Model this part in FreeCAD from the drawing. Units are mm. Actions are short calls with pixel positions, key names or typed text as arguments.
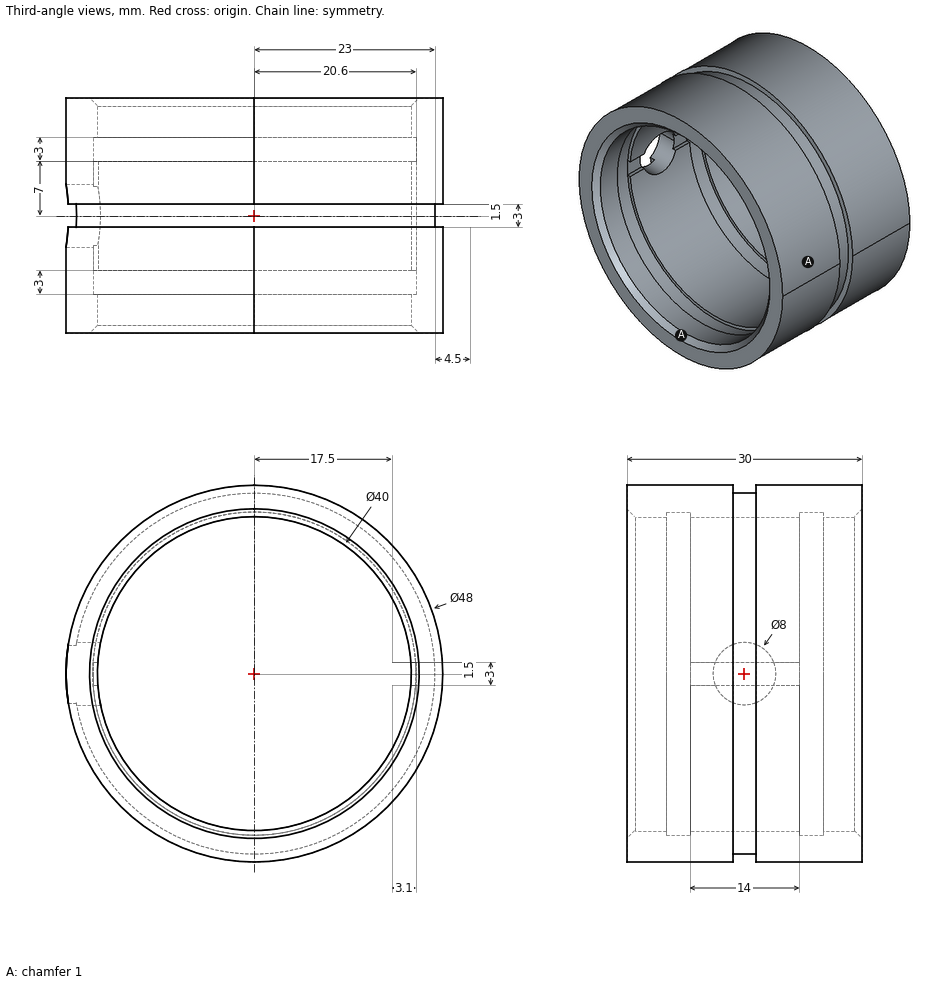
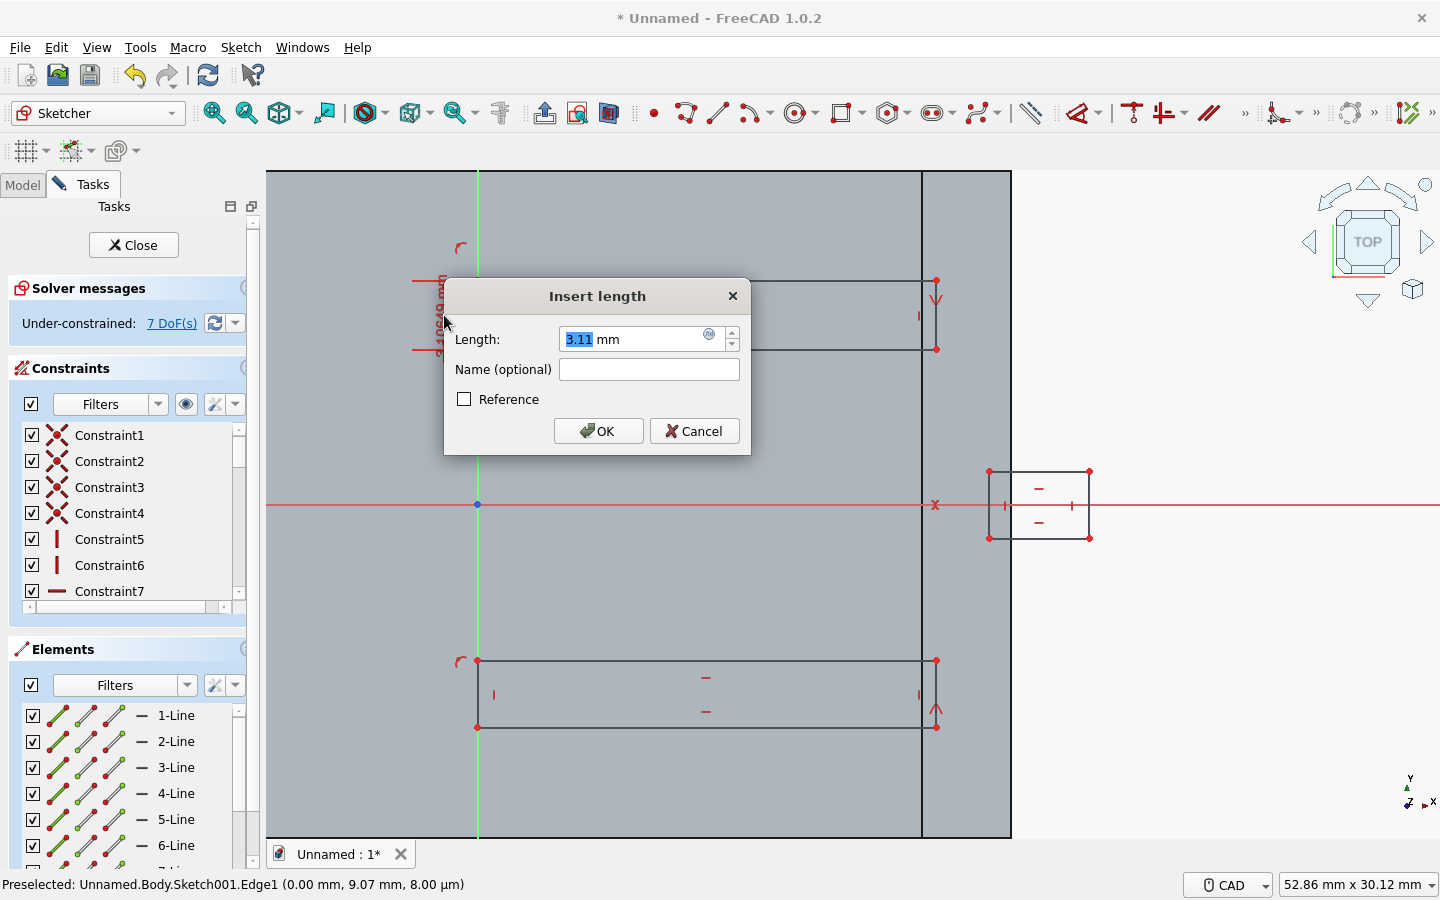
text(3)
key(Return)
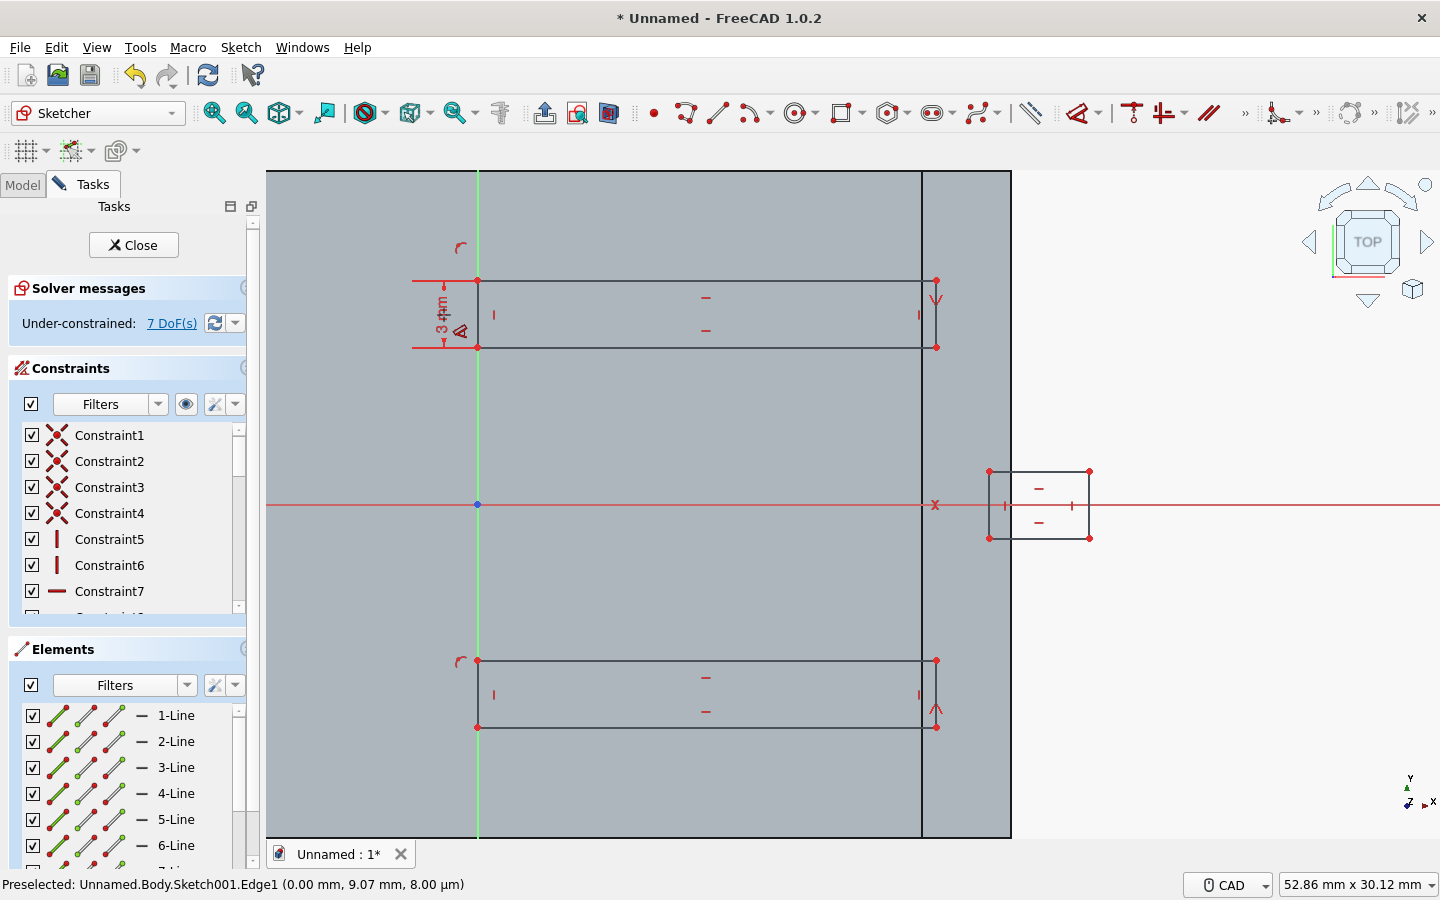
click(478, 681)
click(444, 695)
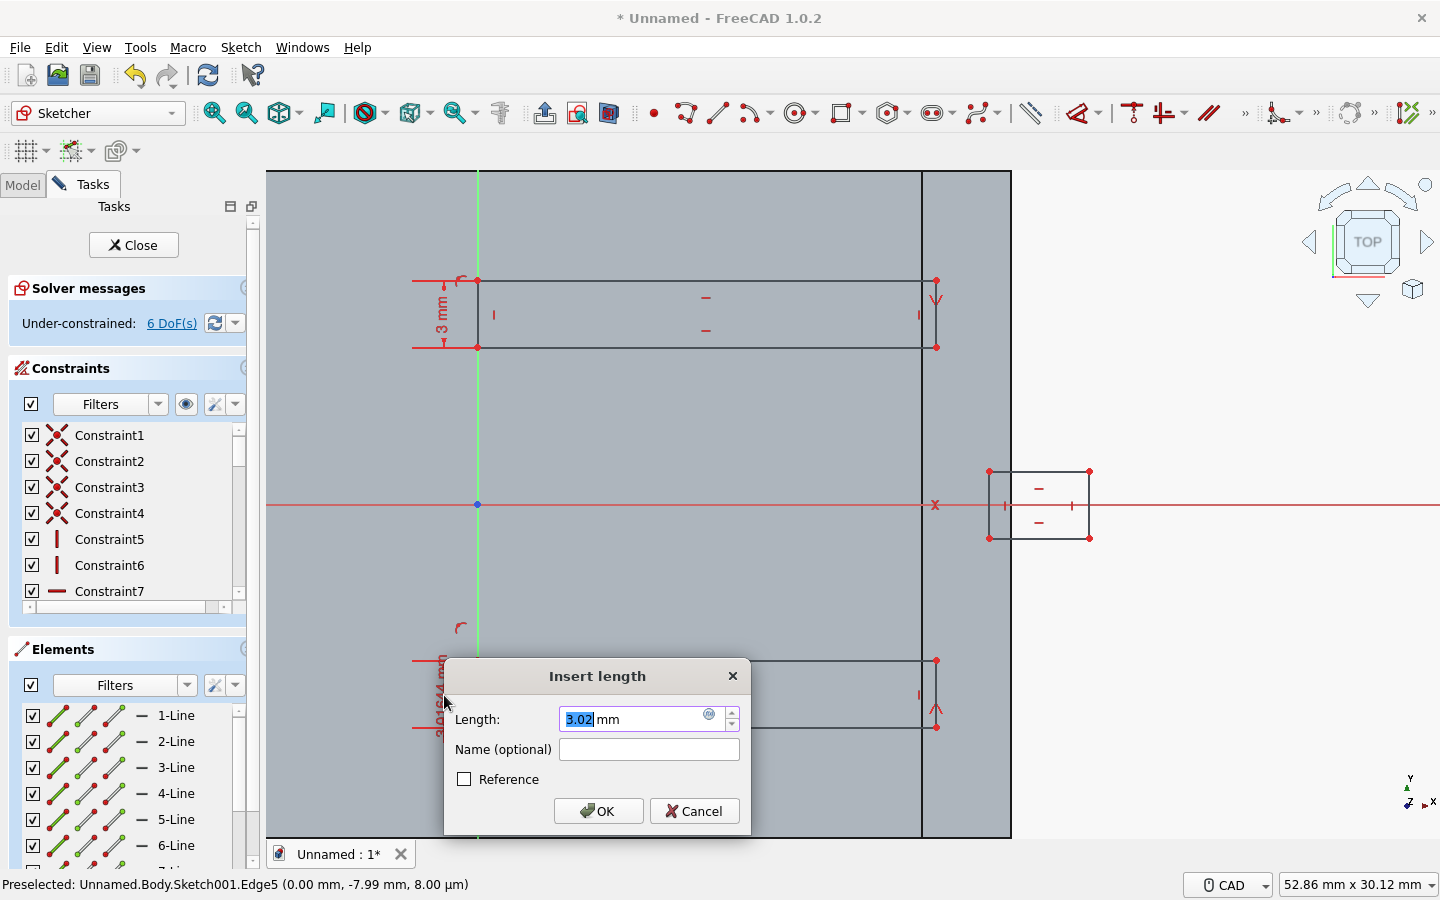
text(3)
key(Return)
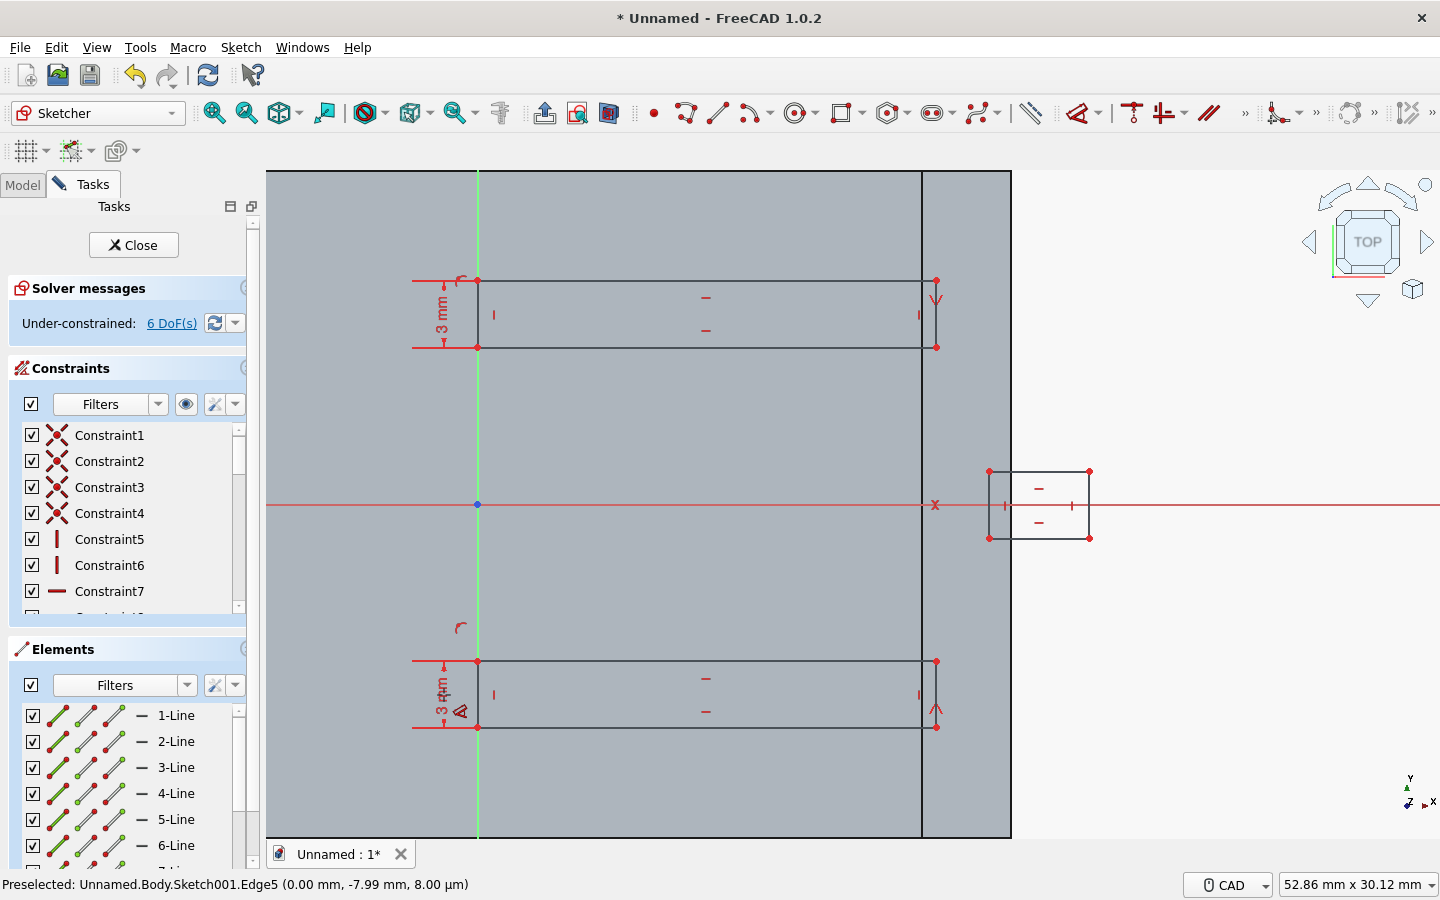
click(989, 492)
click(1023, 490)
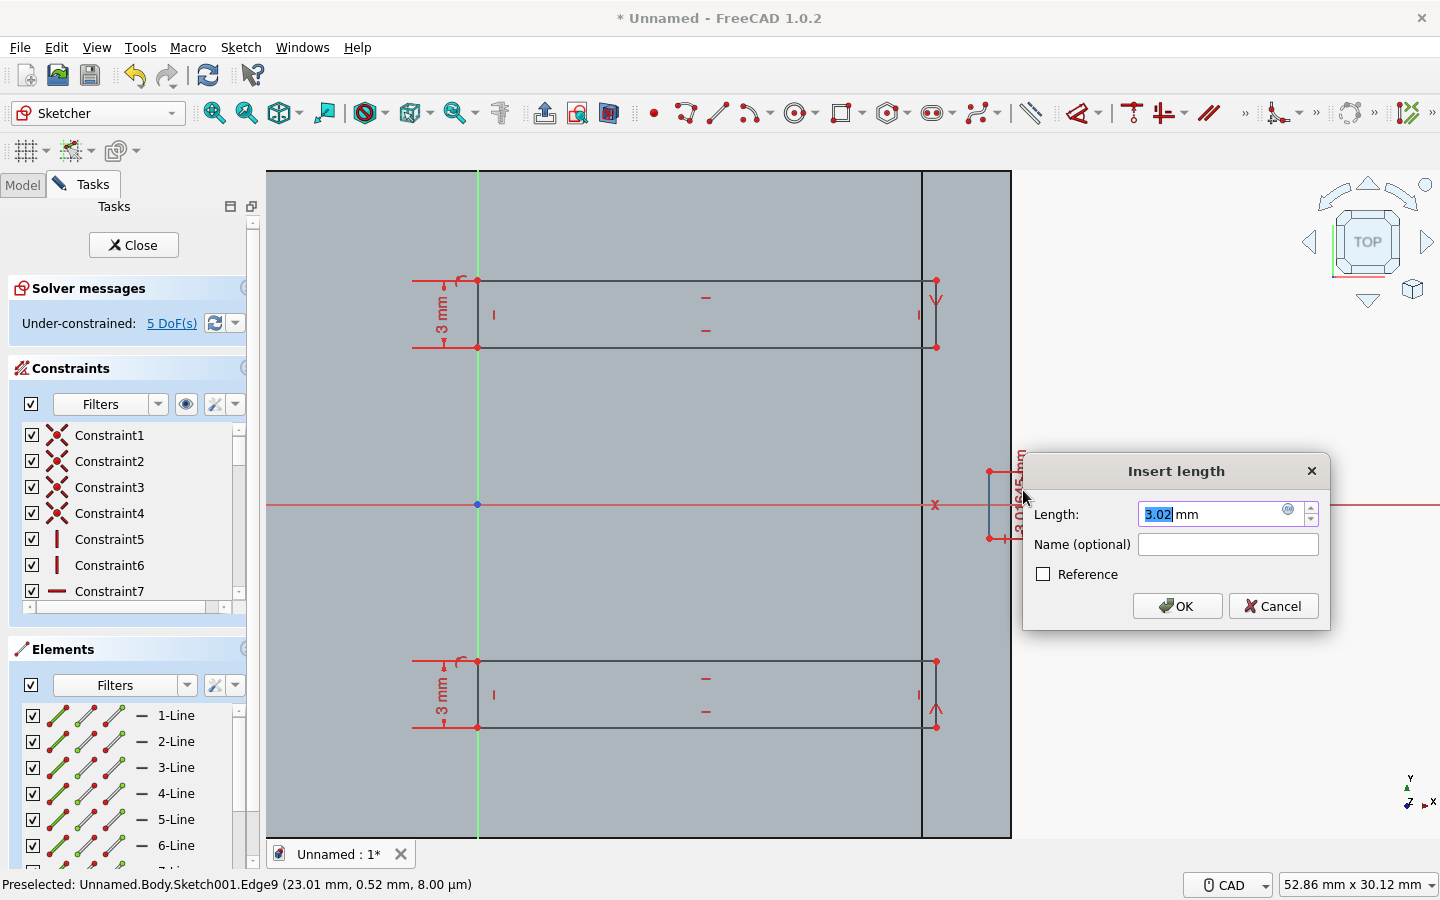
text(3)
key(Return)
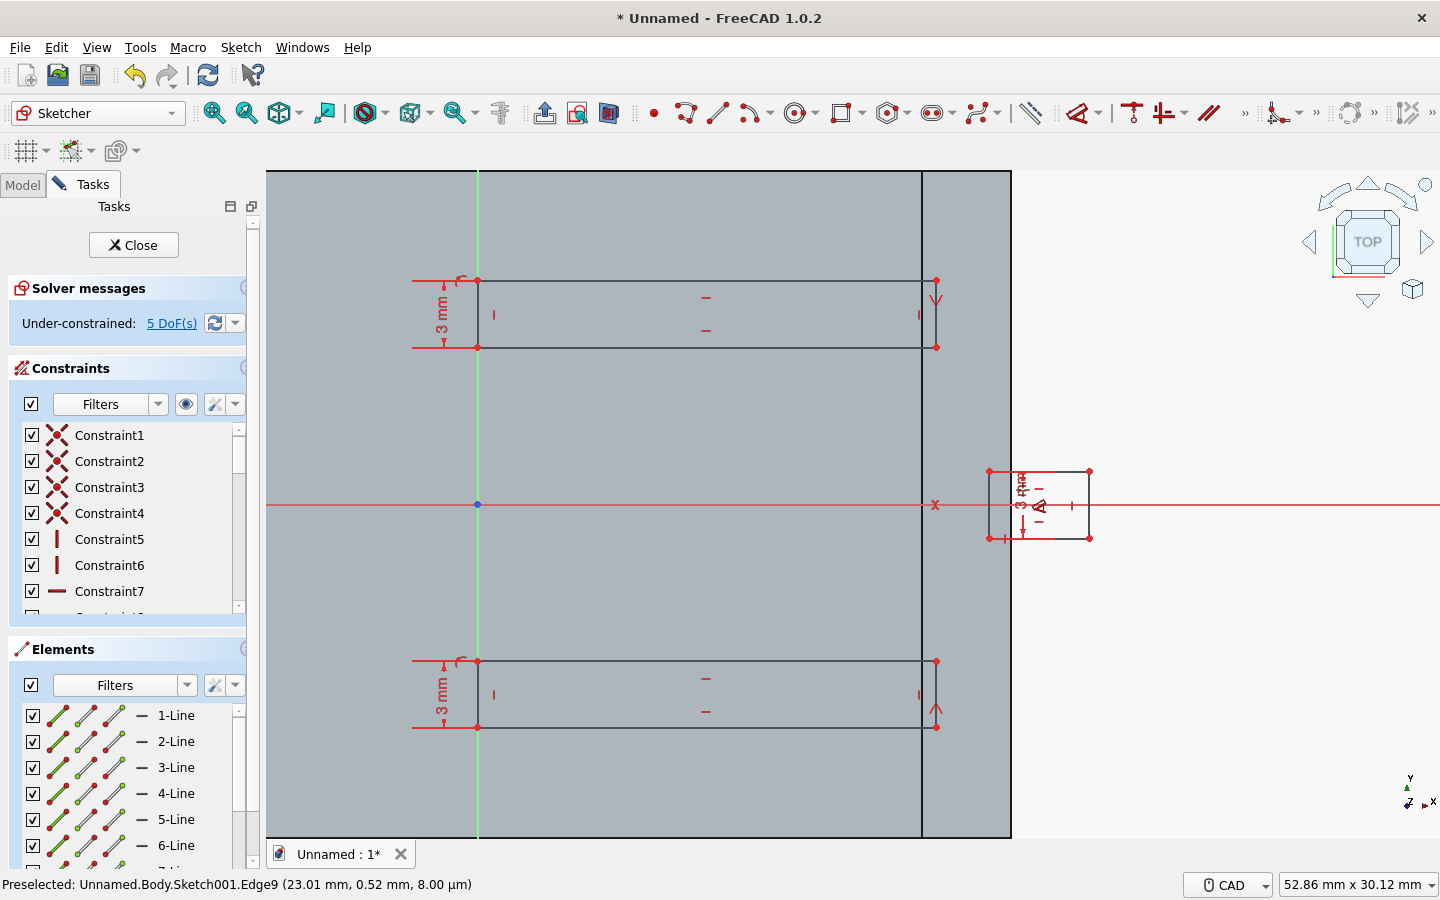
click(478, 348)
click(444, 426)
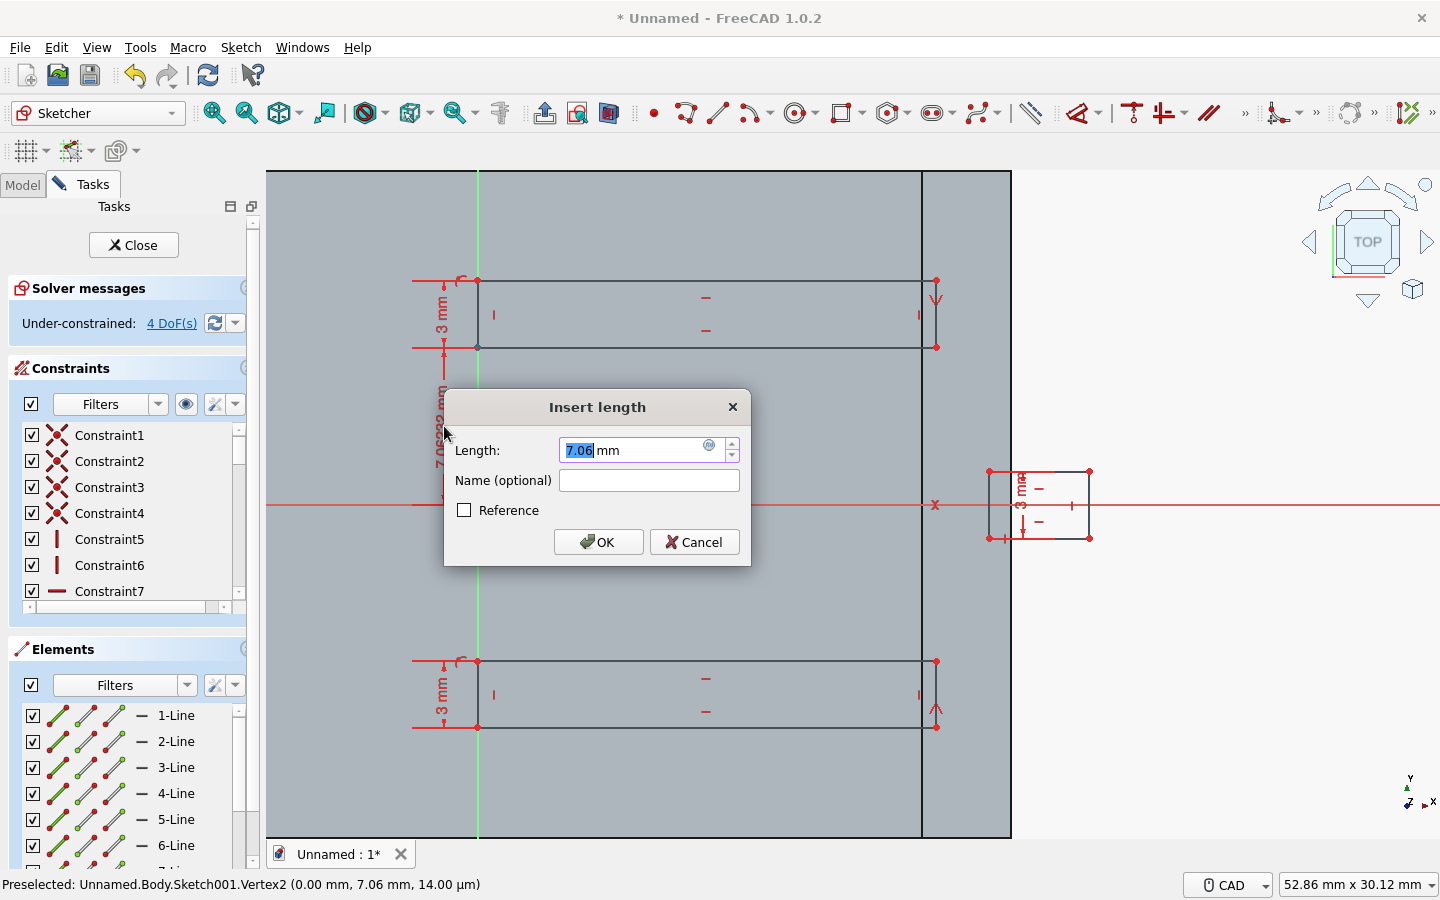
text(7)
key(Return)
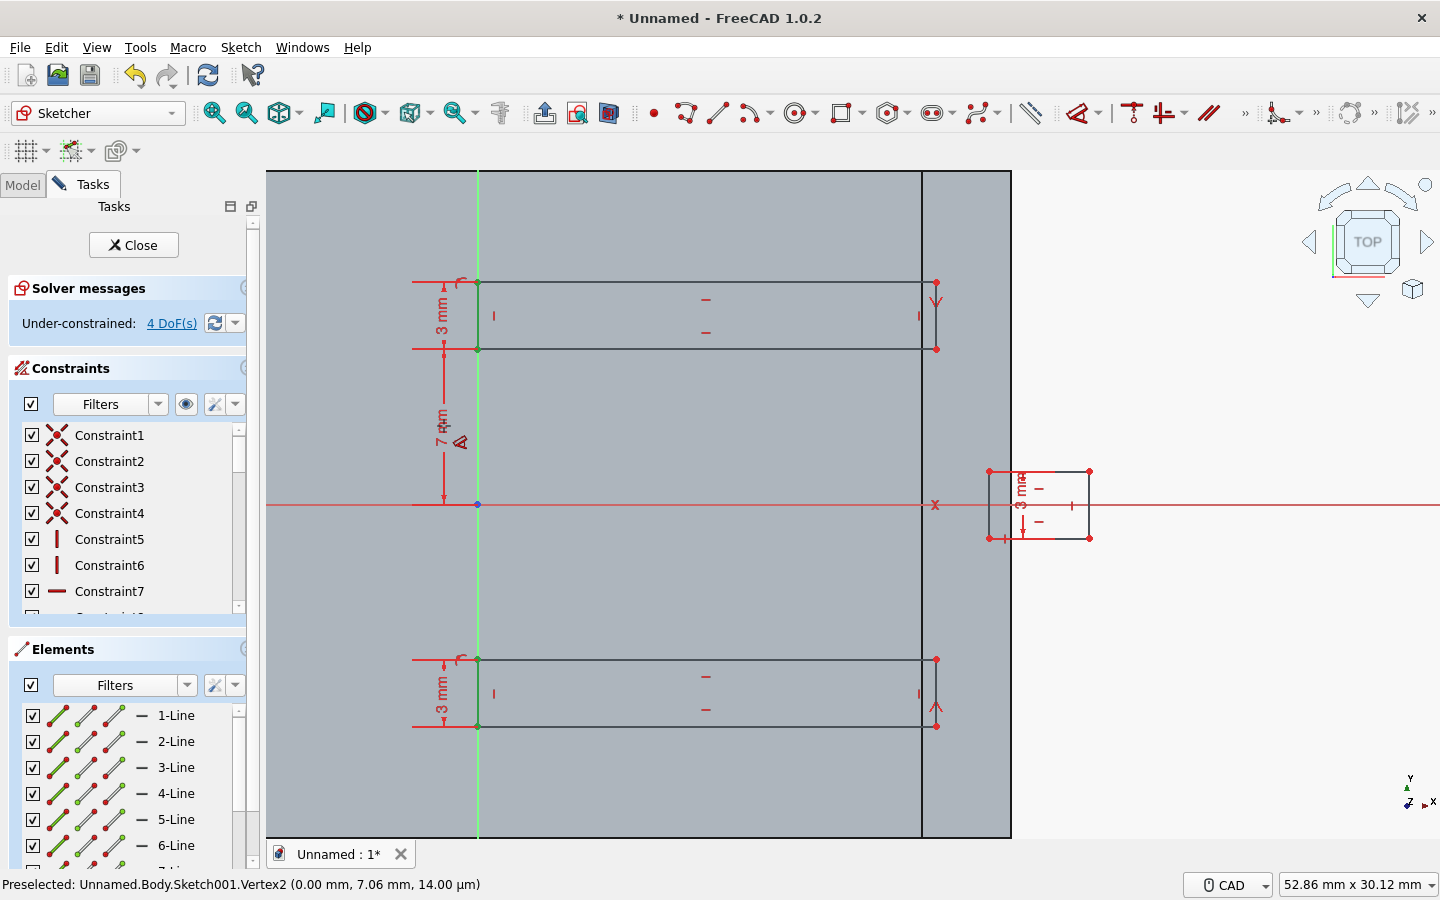
click(1019, 539)
click(1039, 573)